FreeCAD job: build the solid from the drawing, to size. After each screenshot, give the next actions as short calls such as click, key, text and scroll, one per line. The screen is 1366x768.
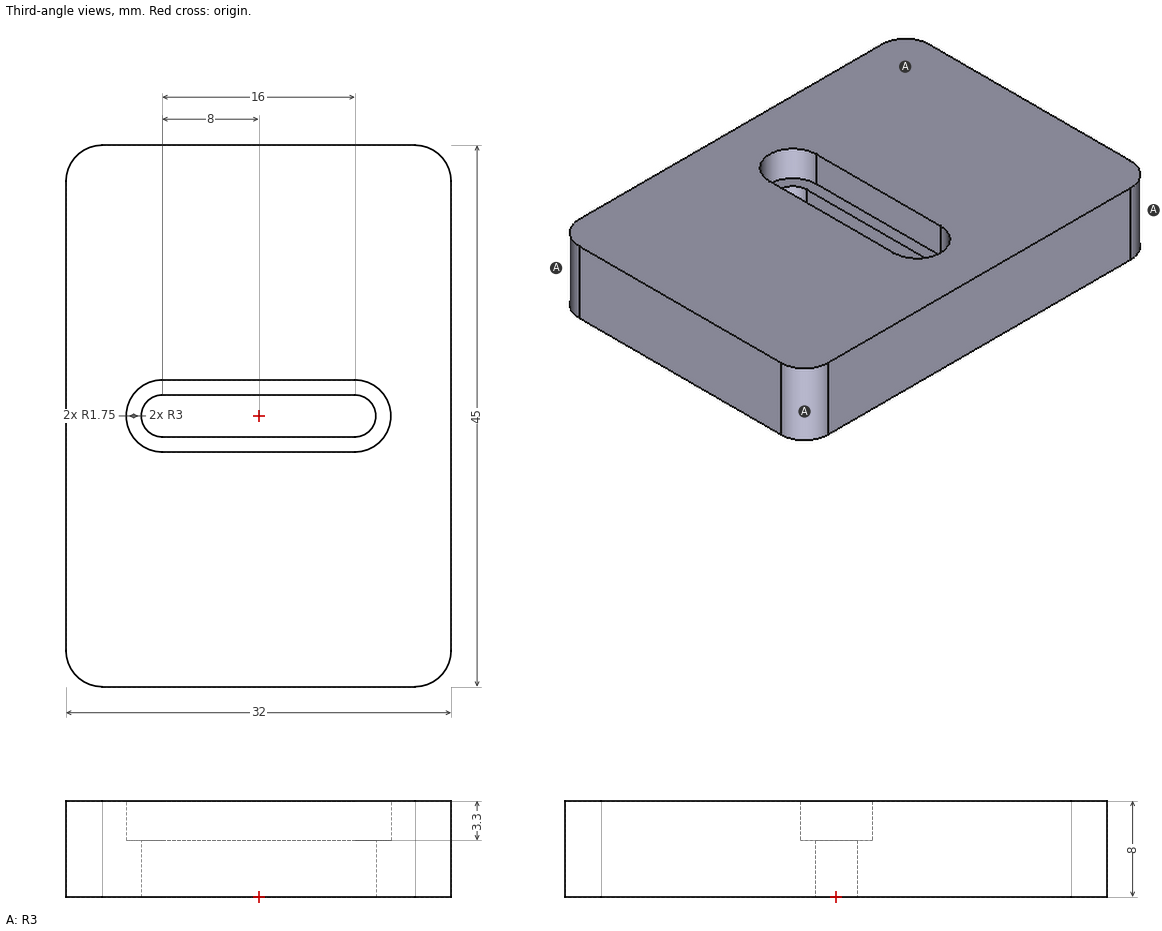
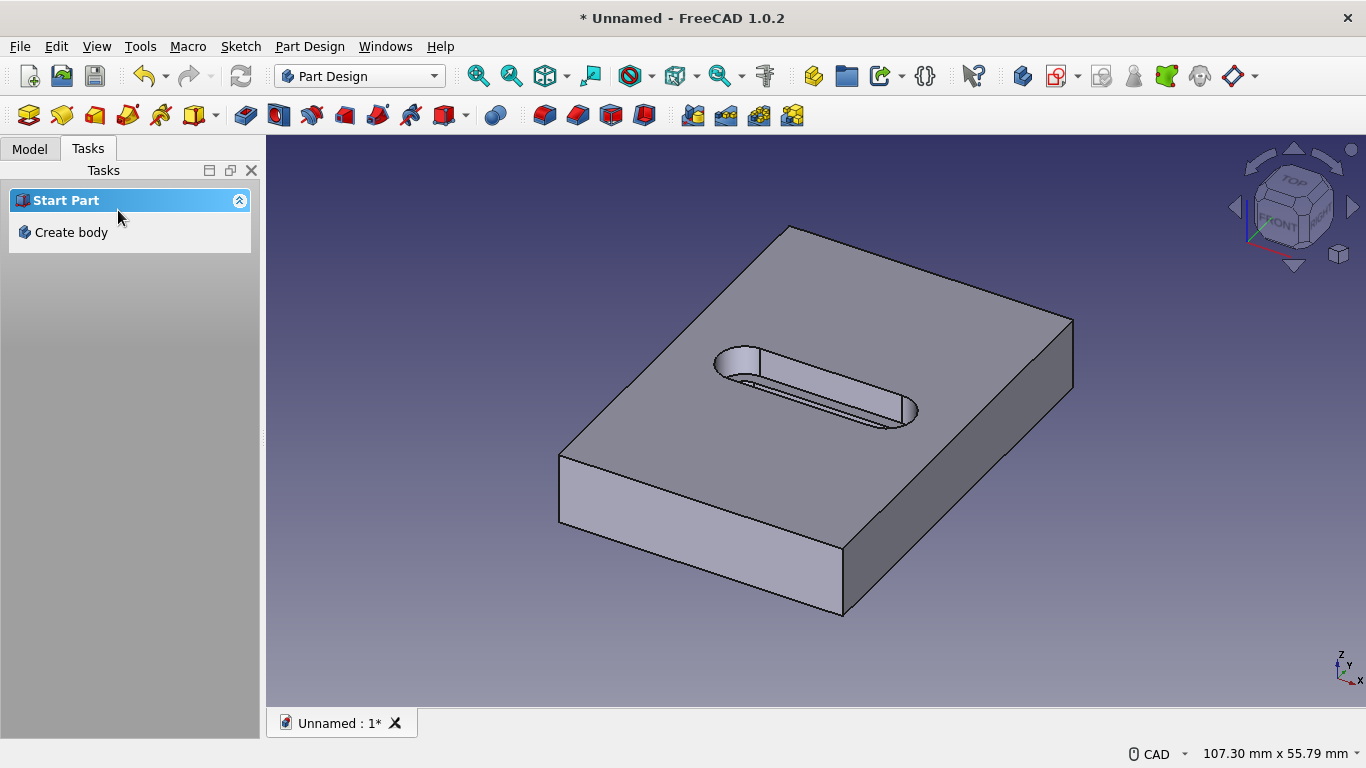
click(843, 582)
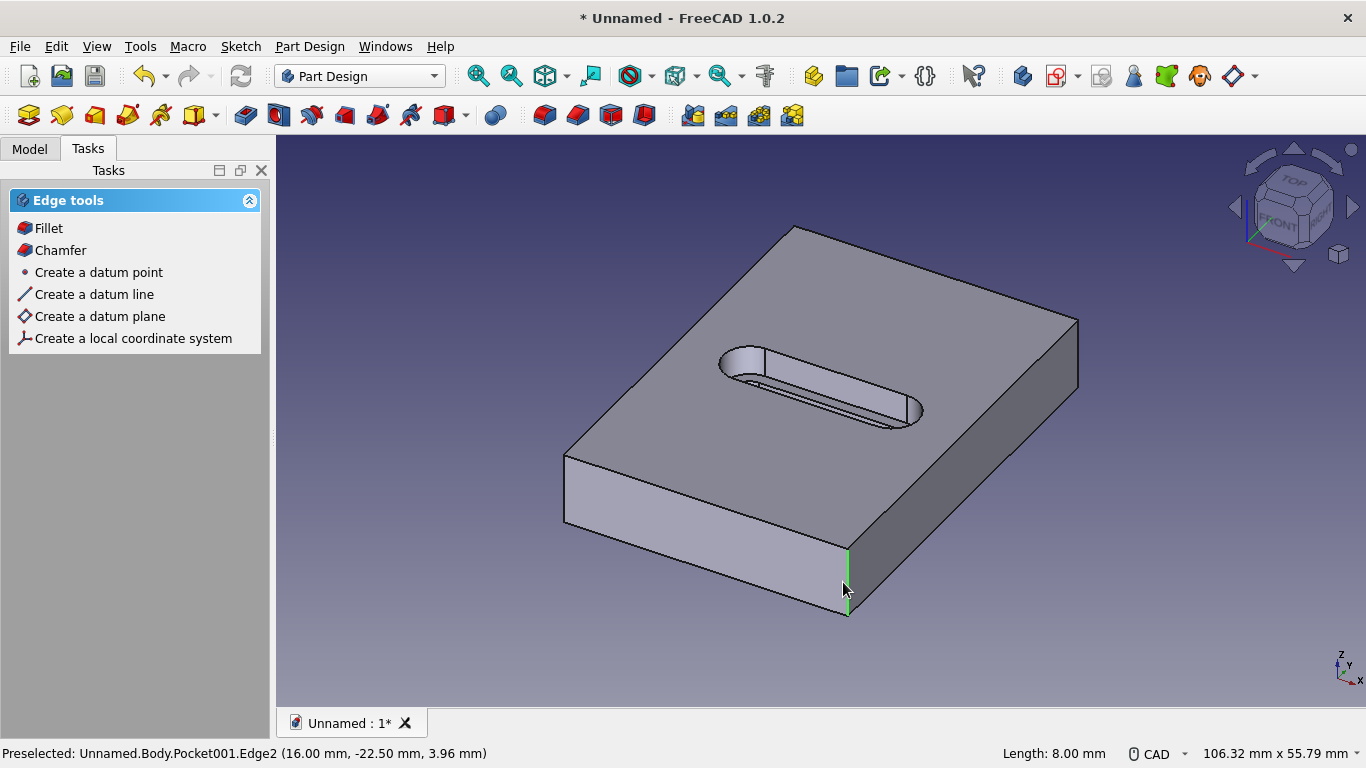
key(0)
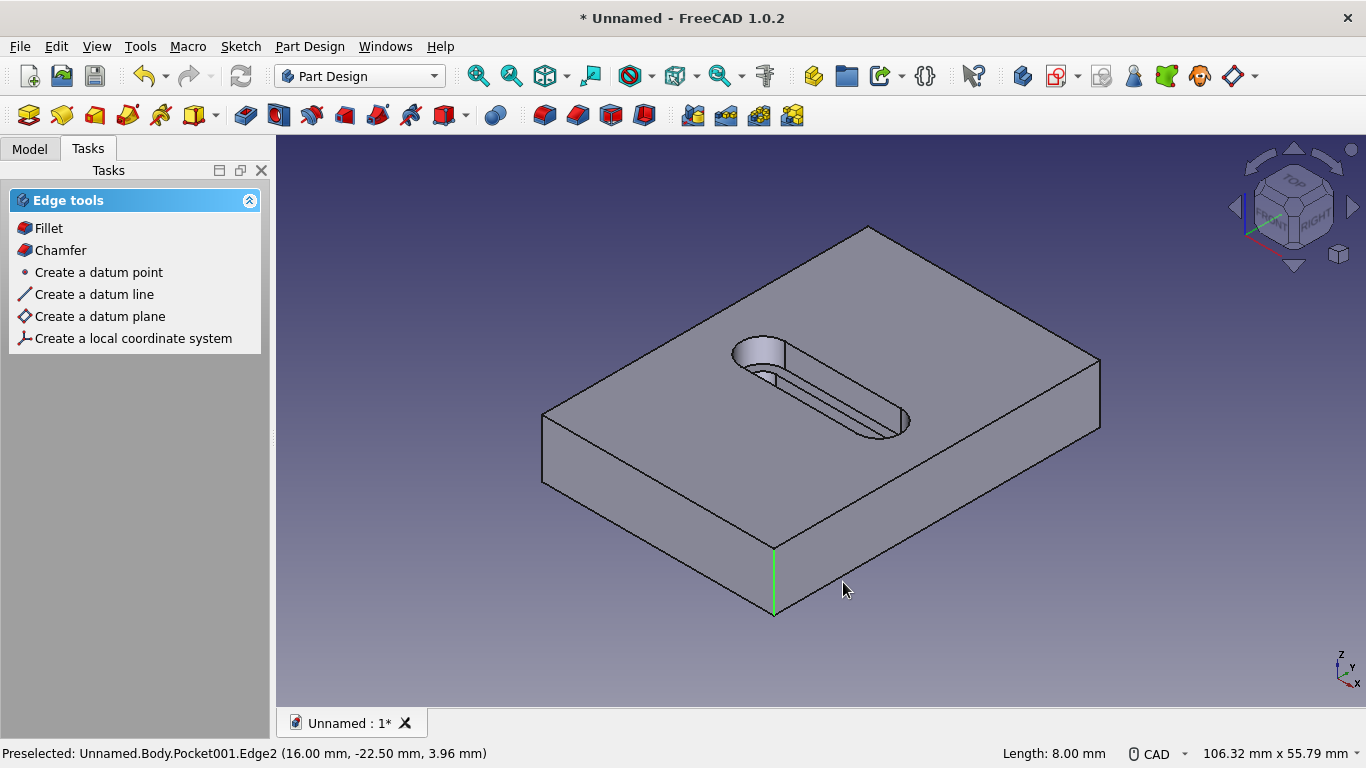
key(2)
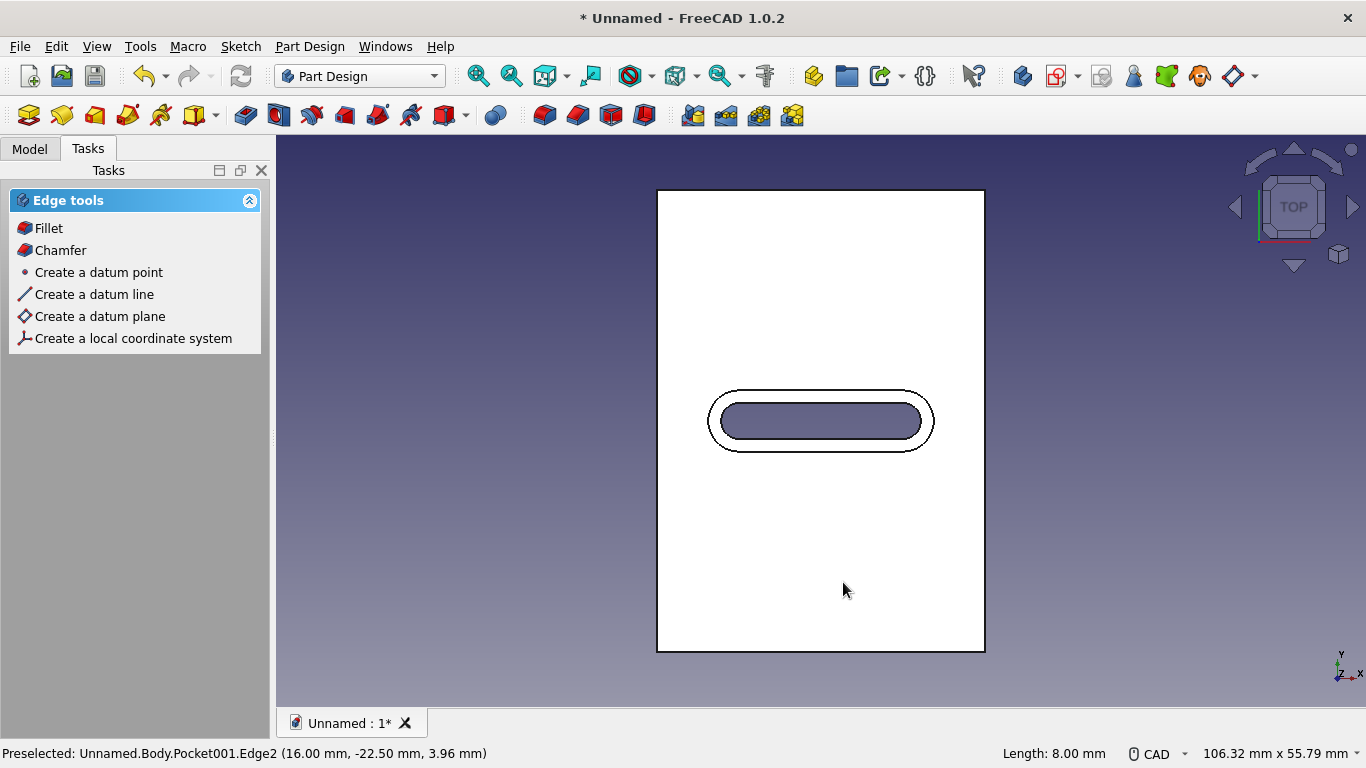
key(1)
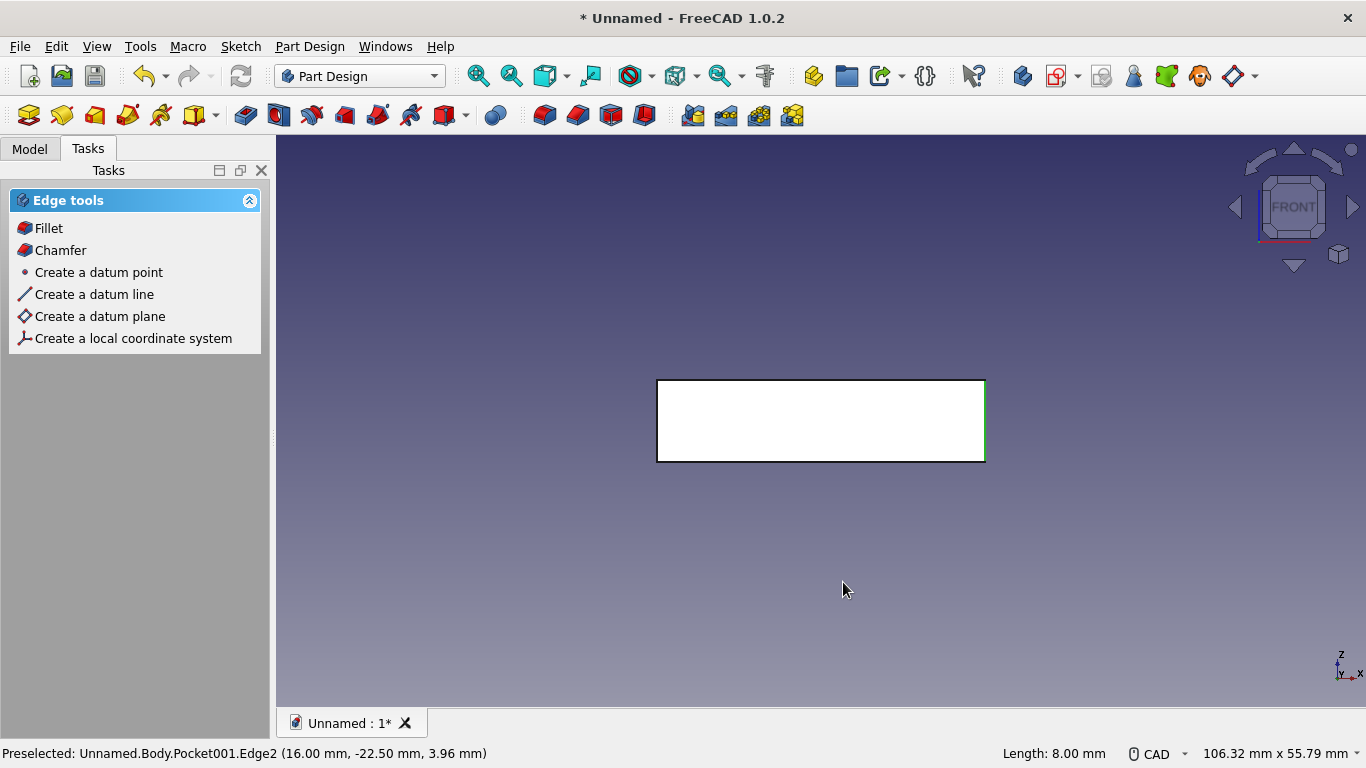
click(479, 76)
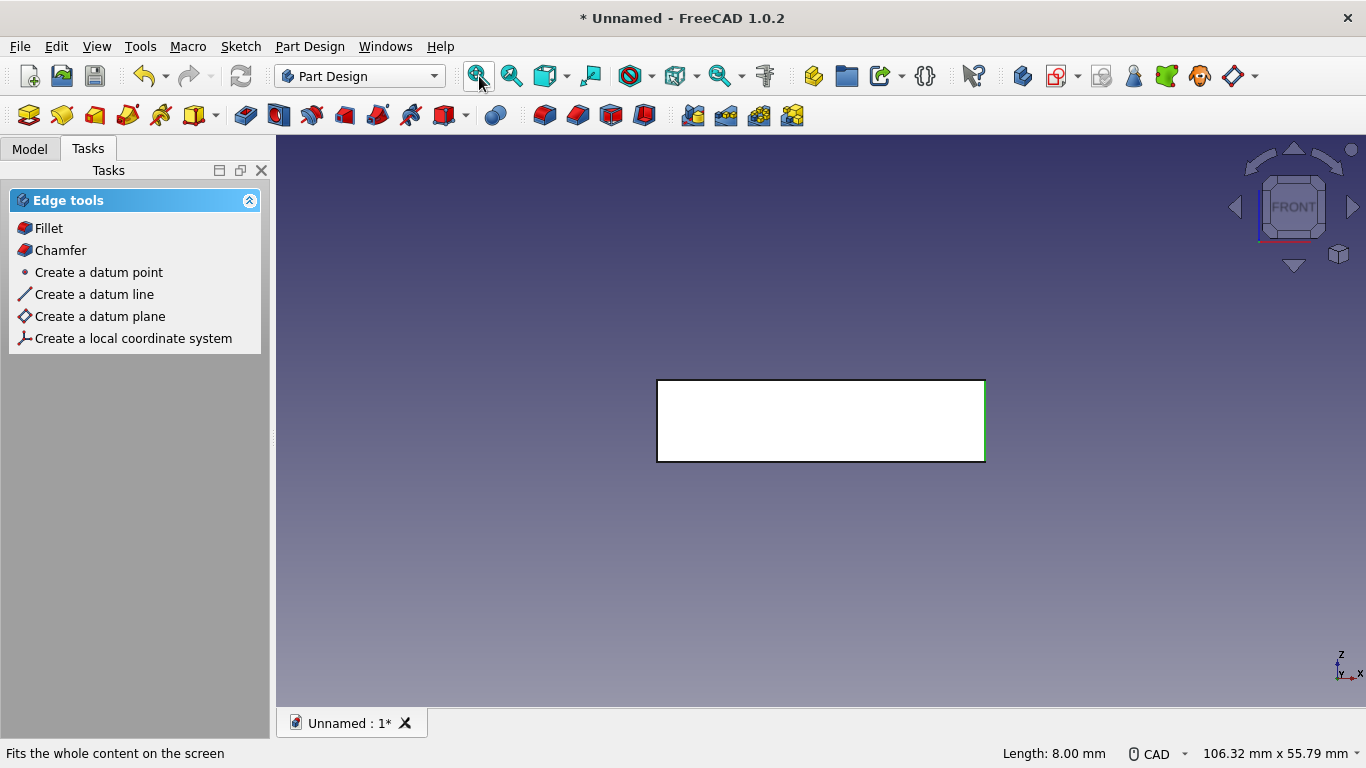
click(657, 420, ctrl)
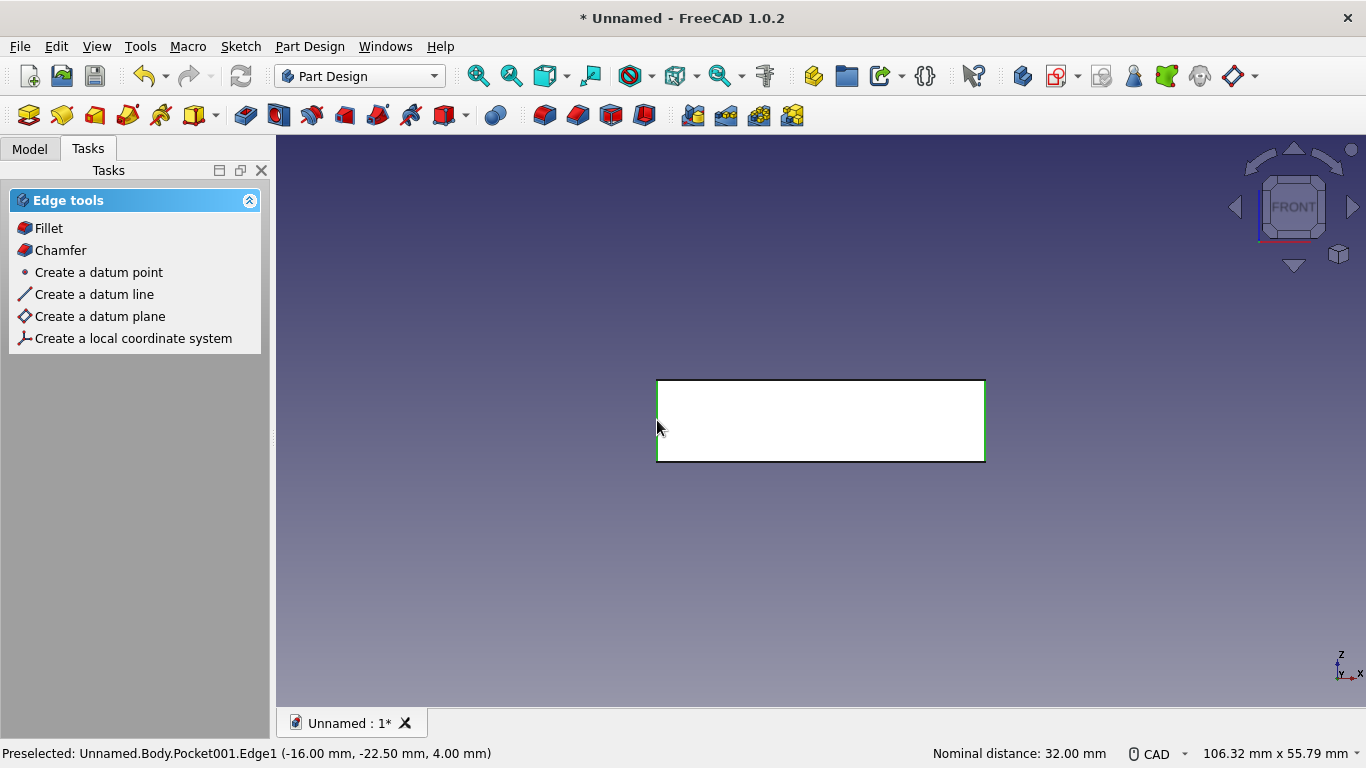
key(3)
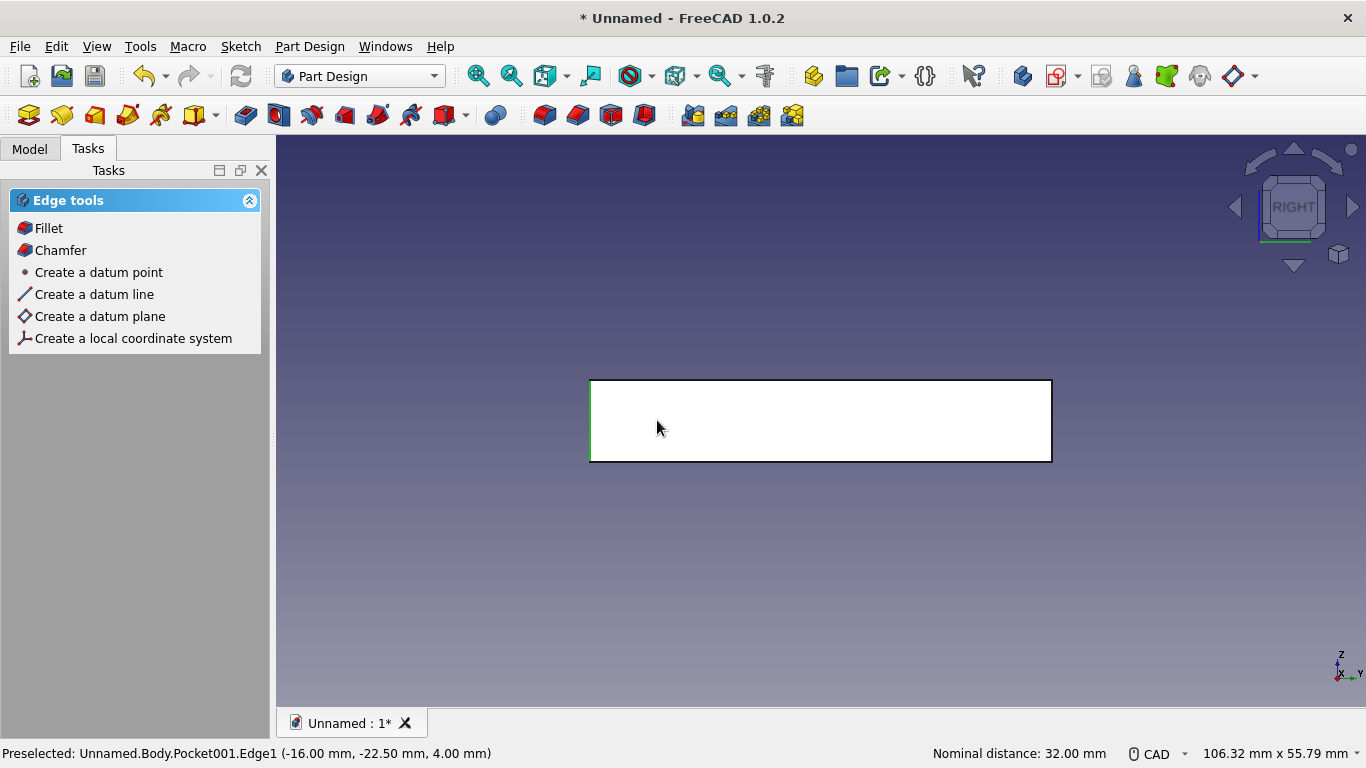
click(479, 76)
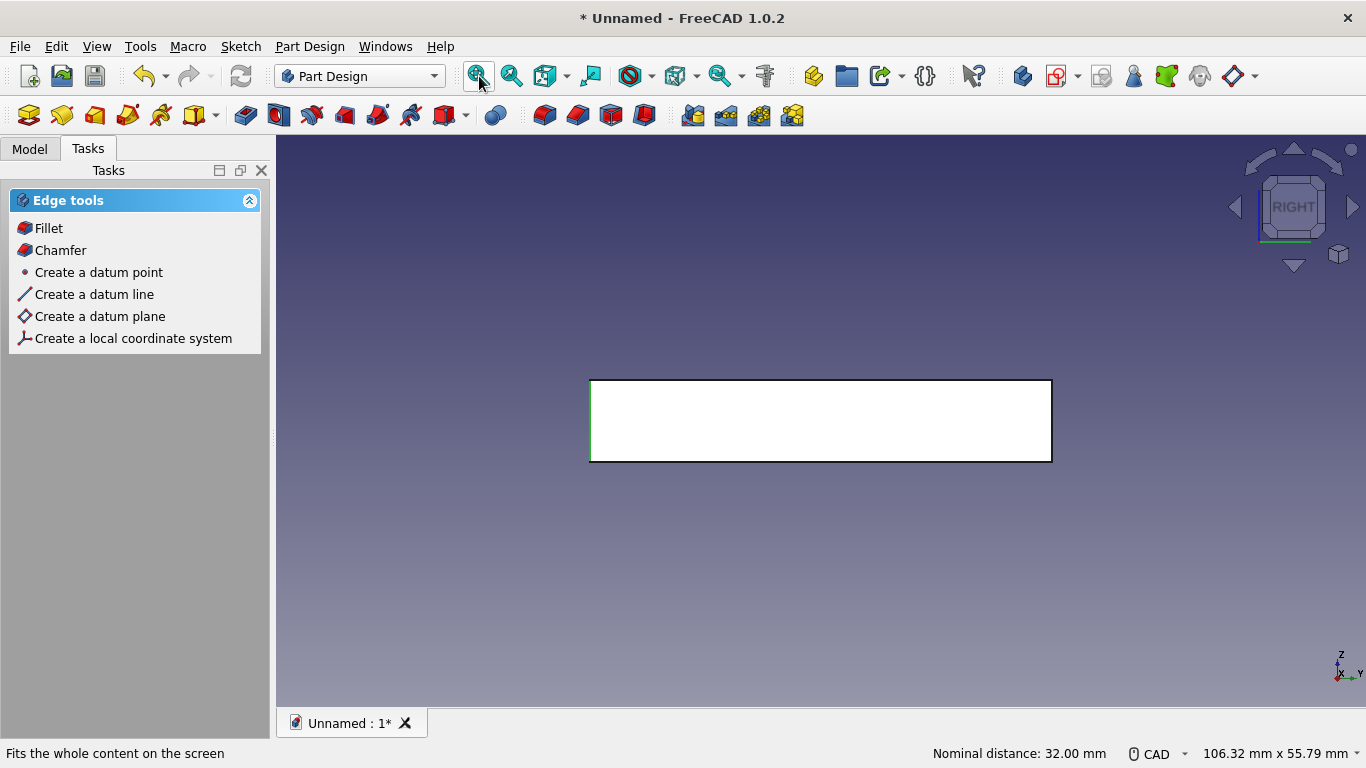
click(1052, 420, ctrl)